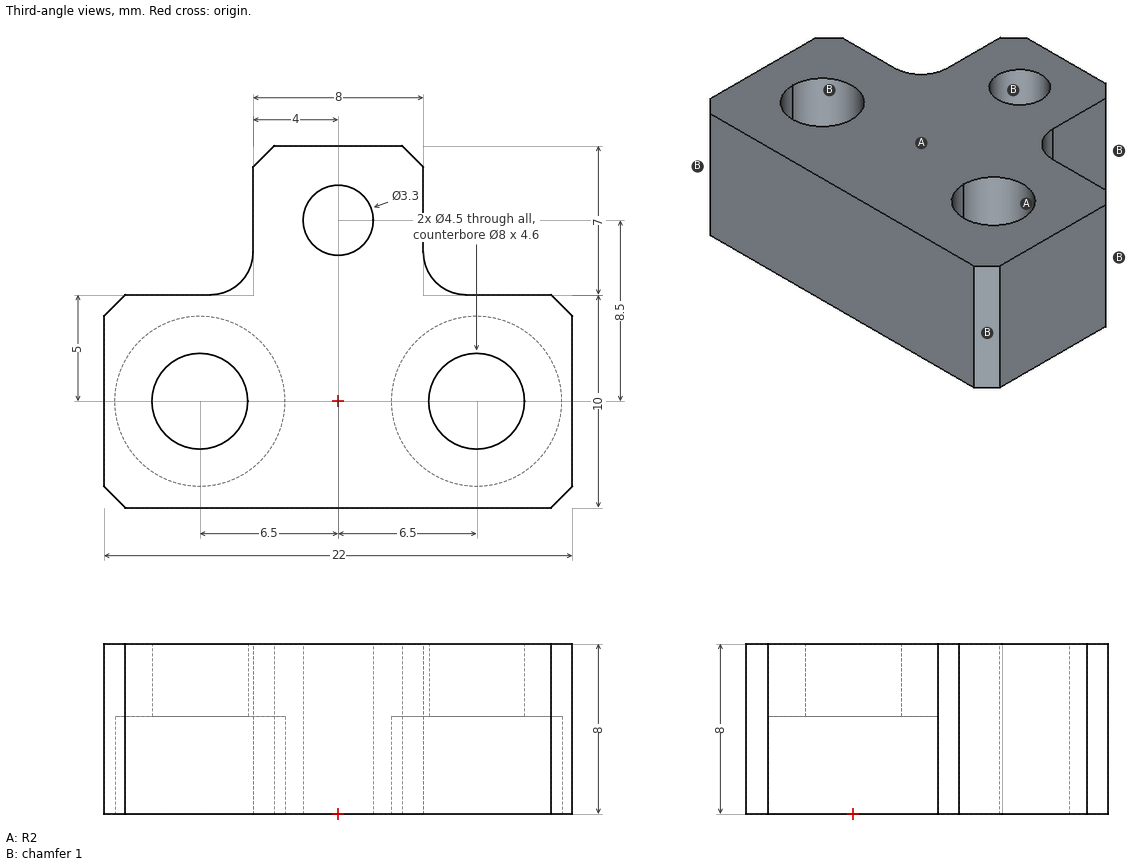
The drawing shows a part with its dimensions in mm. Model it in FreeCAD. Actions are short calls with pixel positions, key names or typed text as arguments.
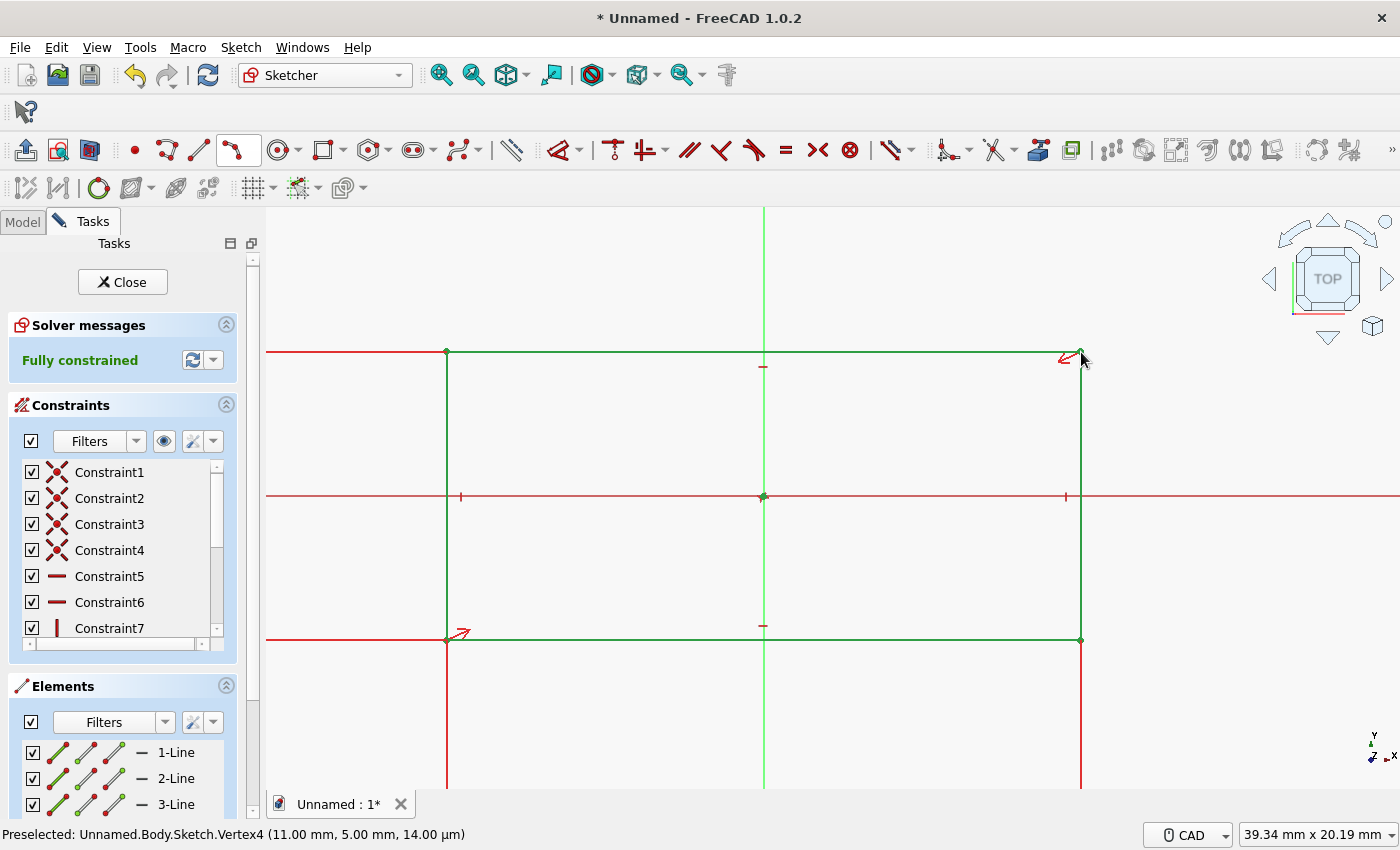
click(123, 282)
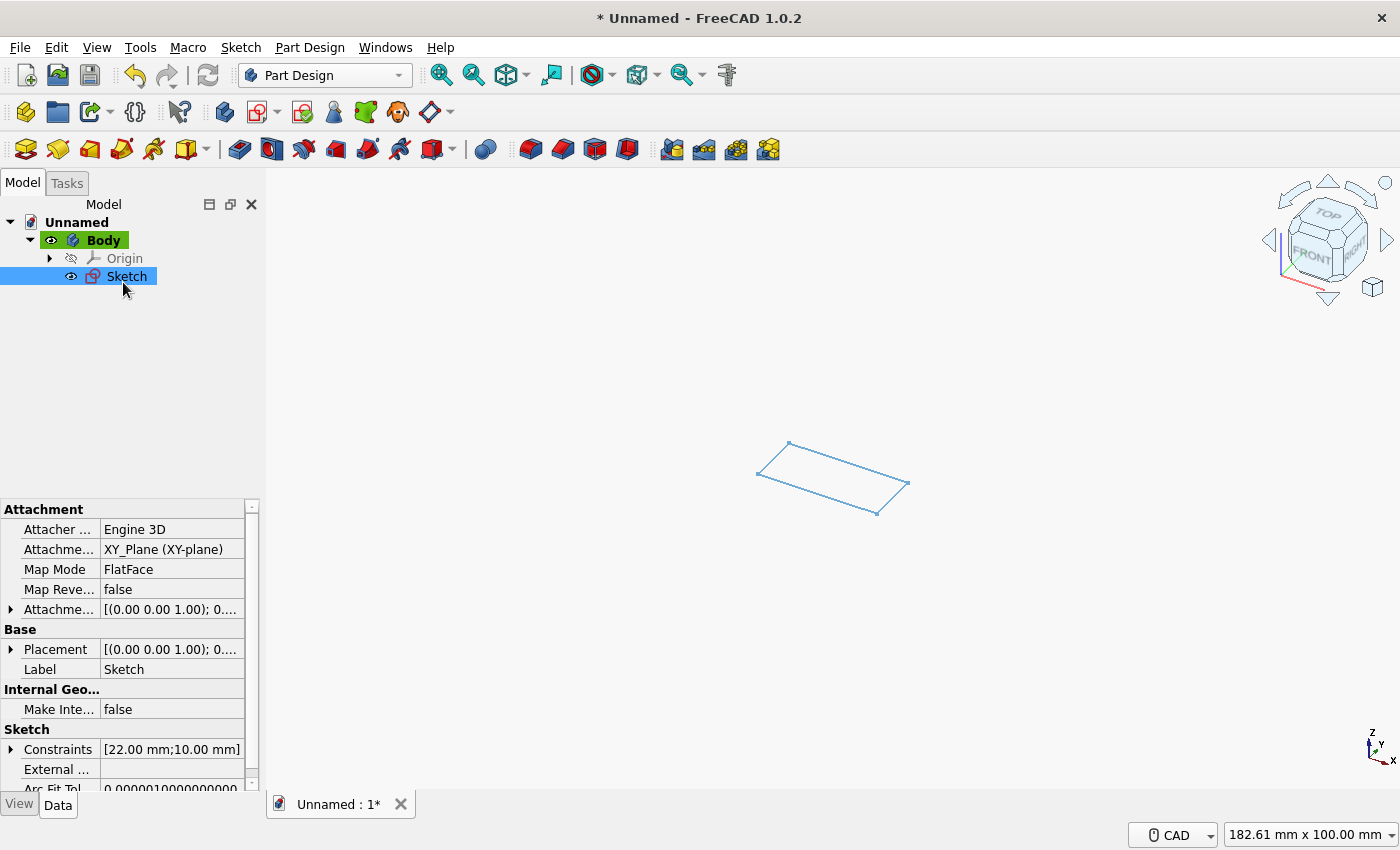
click(26, 150)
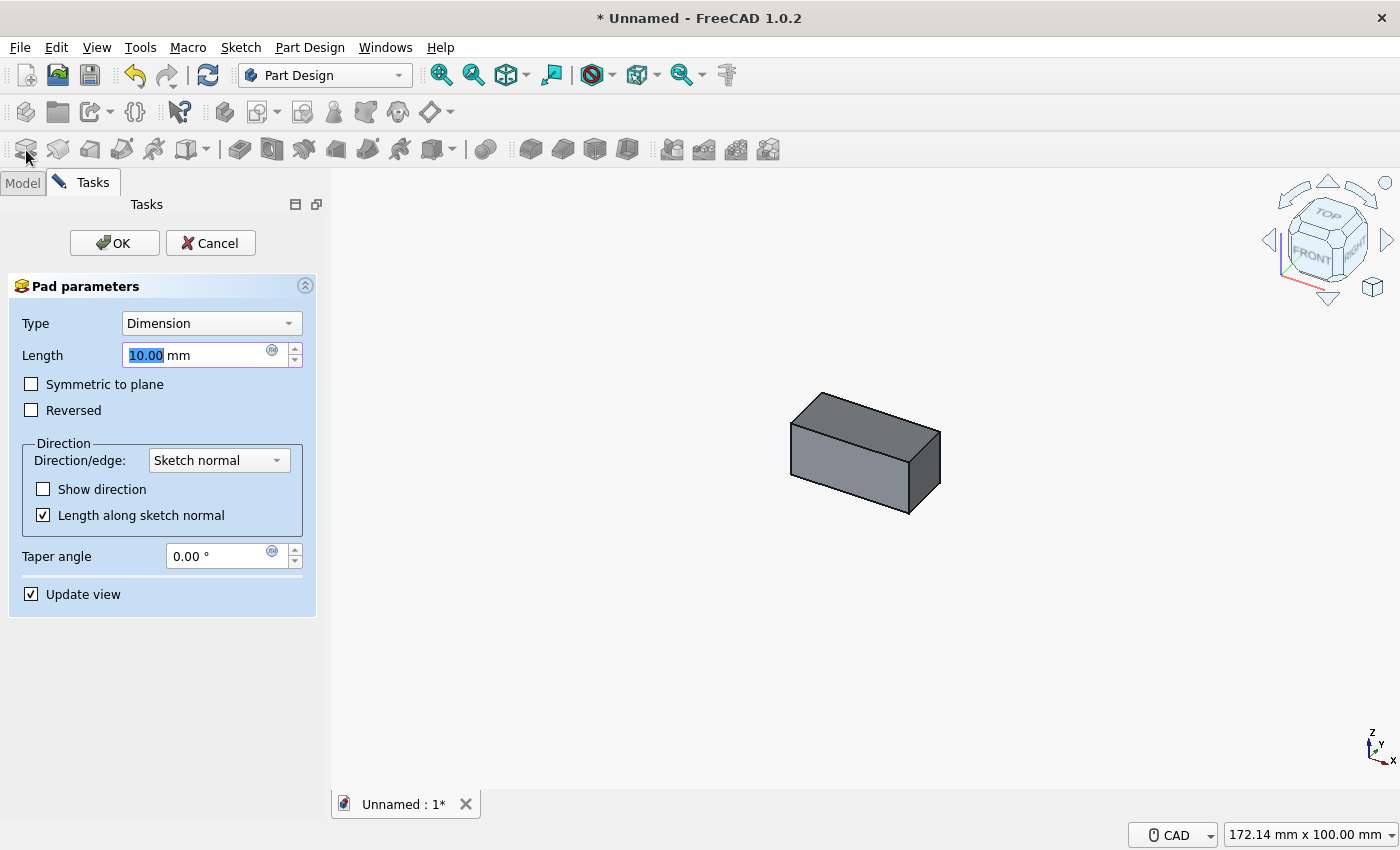
text(8)
key(Tab)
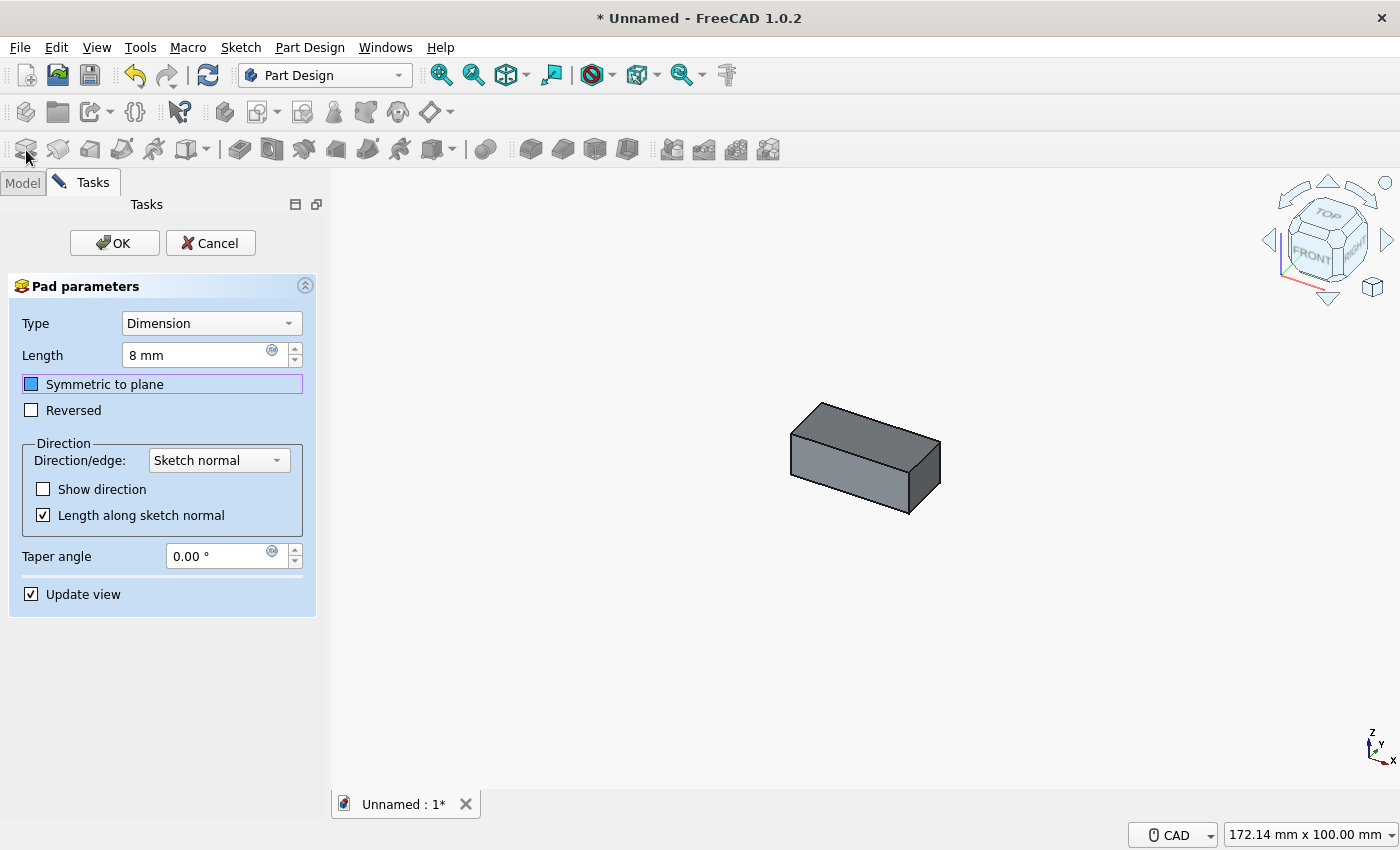
click(115, 243)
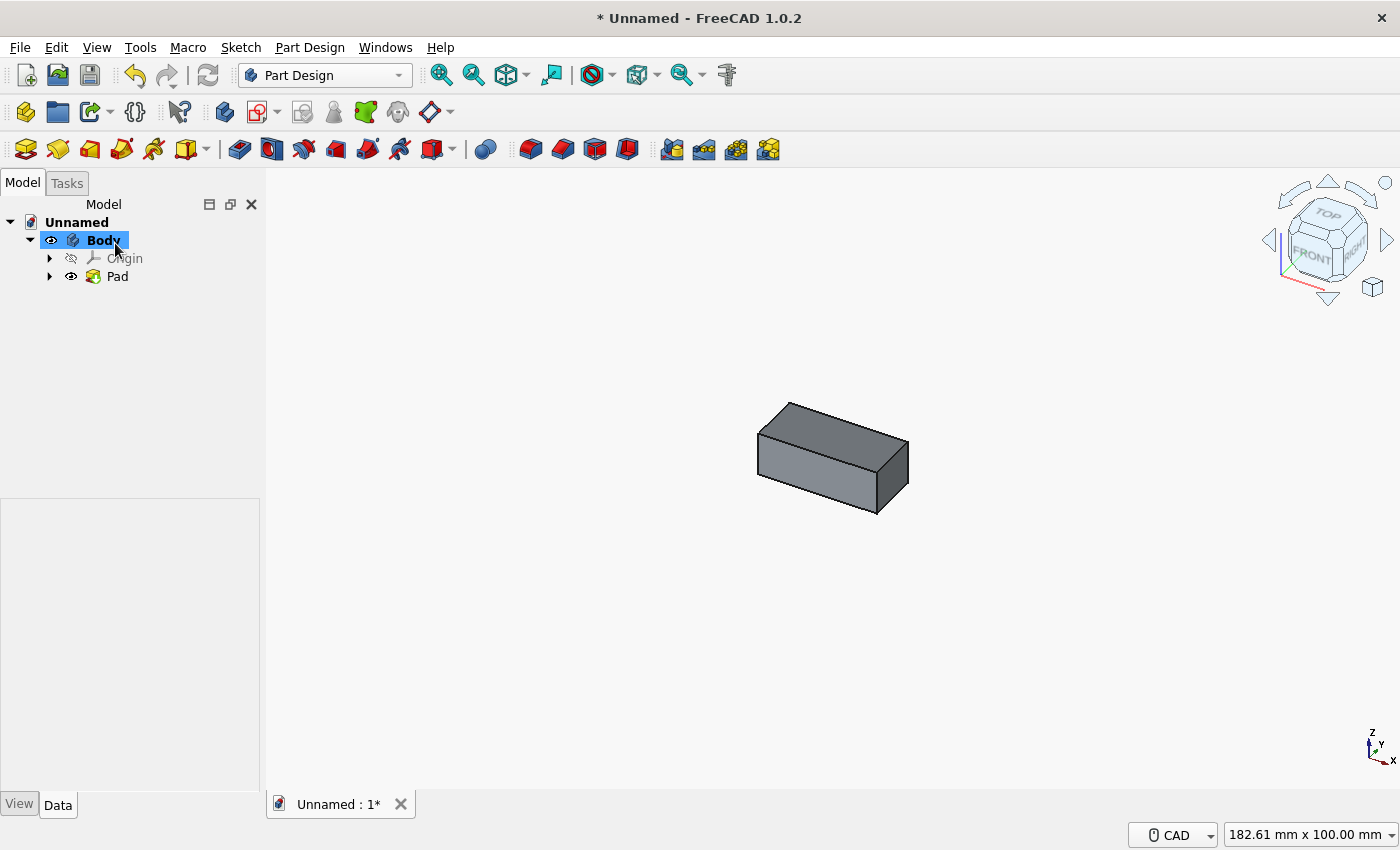
click(442, 76)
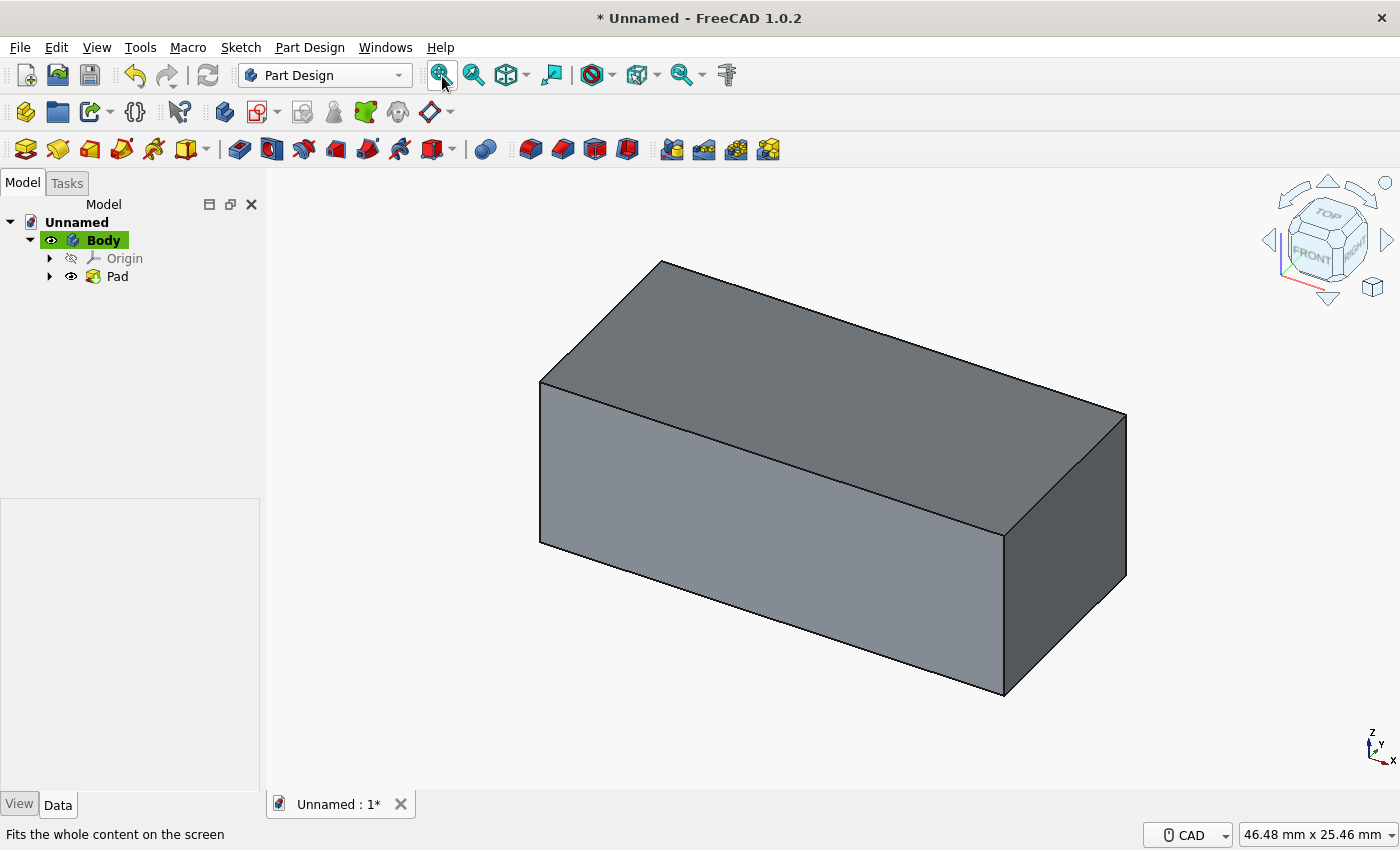
key(5)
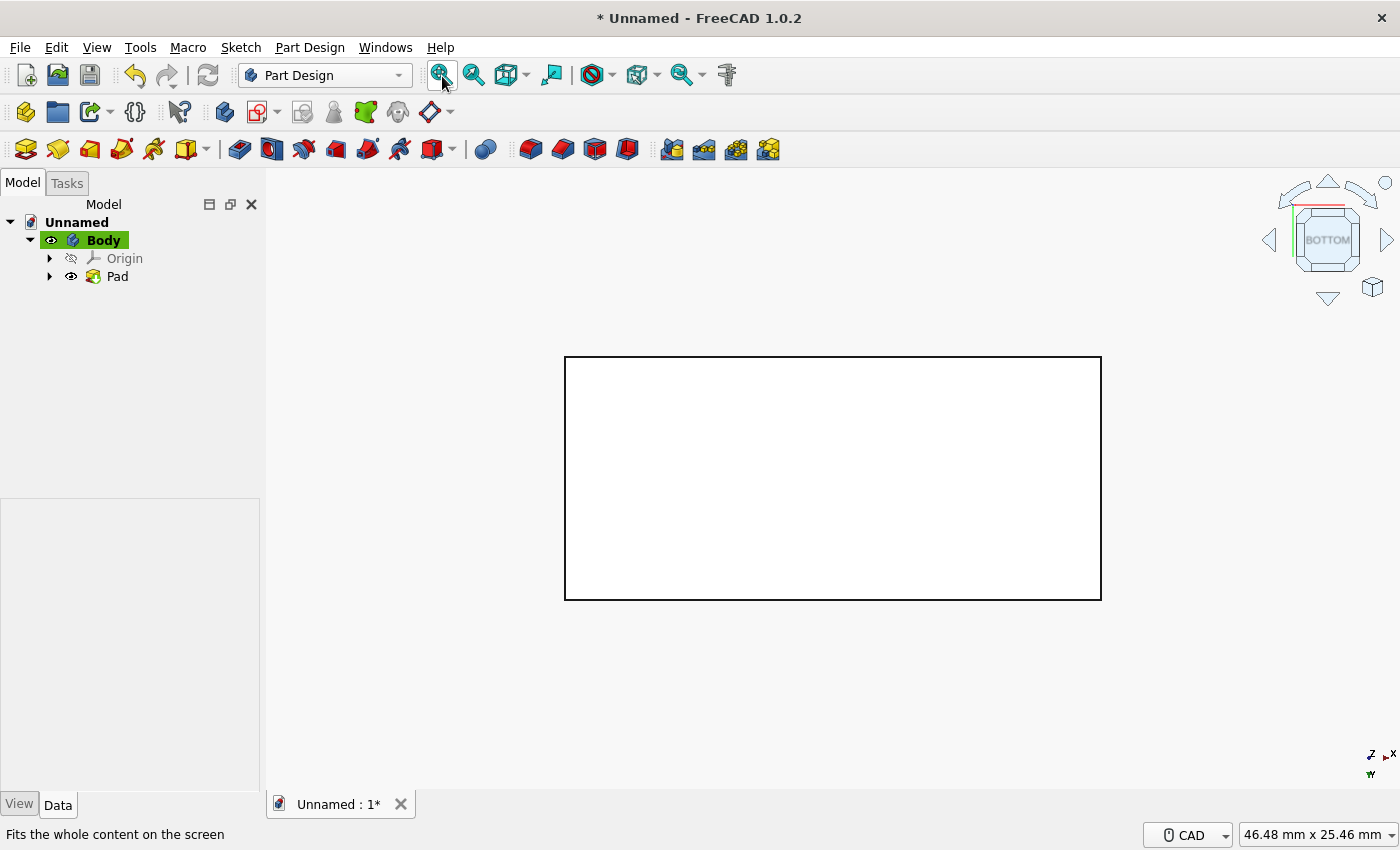
click(910, 477)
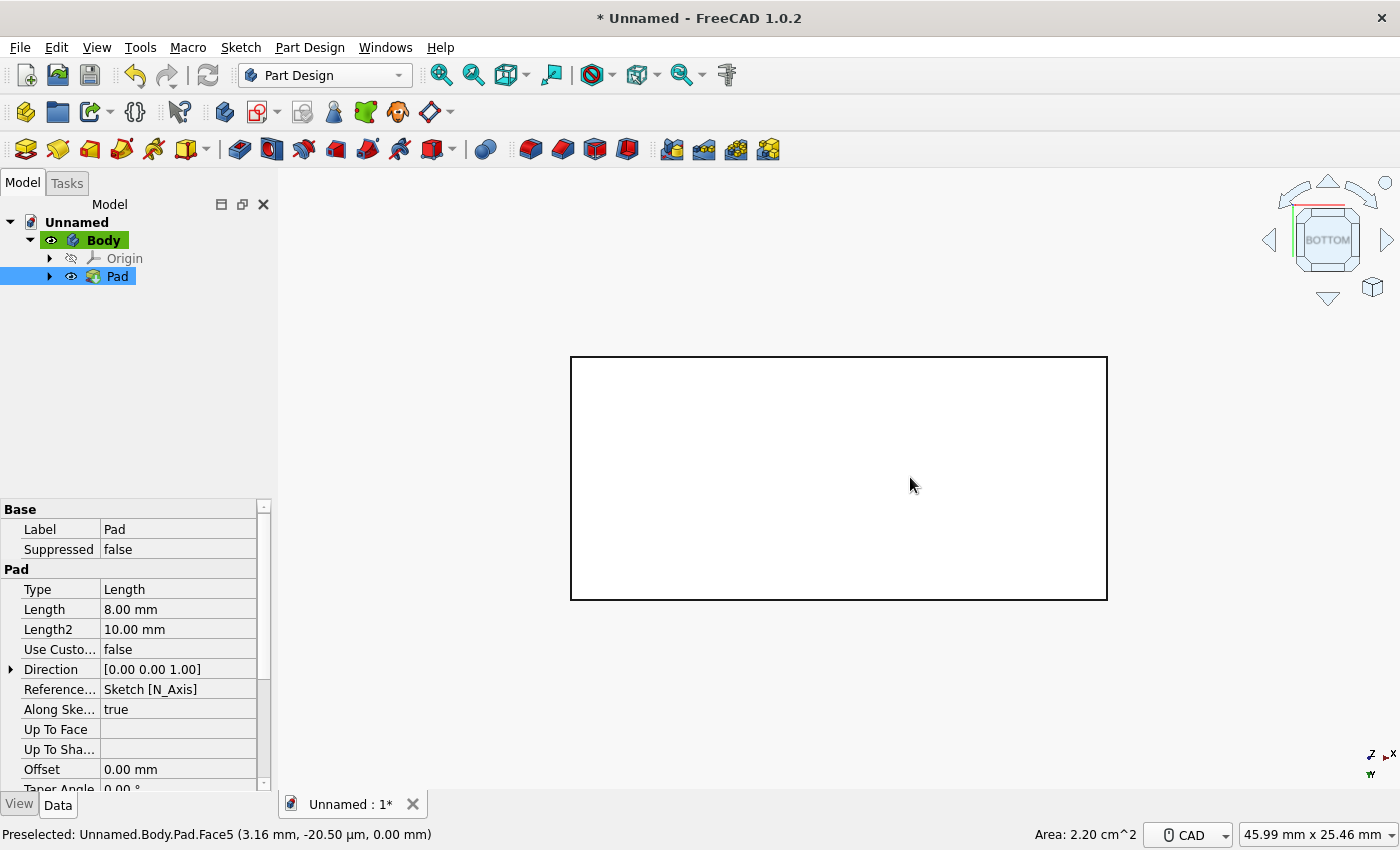
click(258, 112)